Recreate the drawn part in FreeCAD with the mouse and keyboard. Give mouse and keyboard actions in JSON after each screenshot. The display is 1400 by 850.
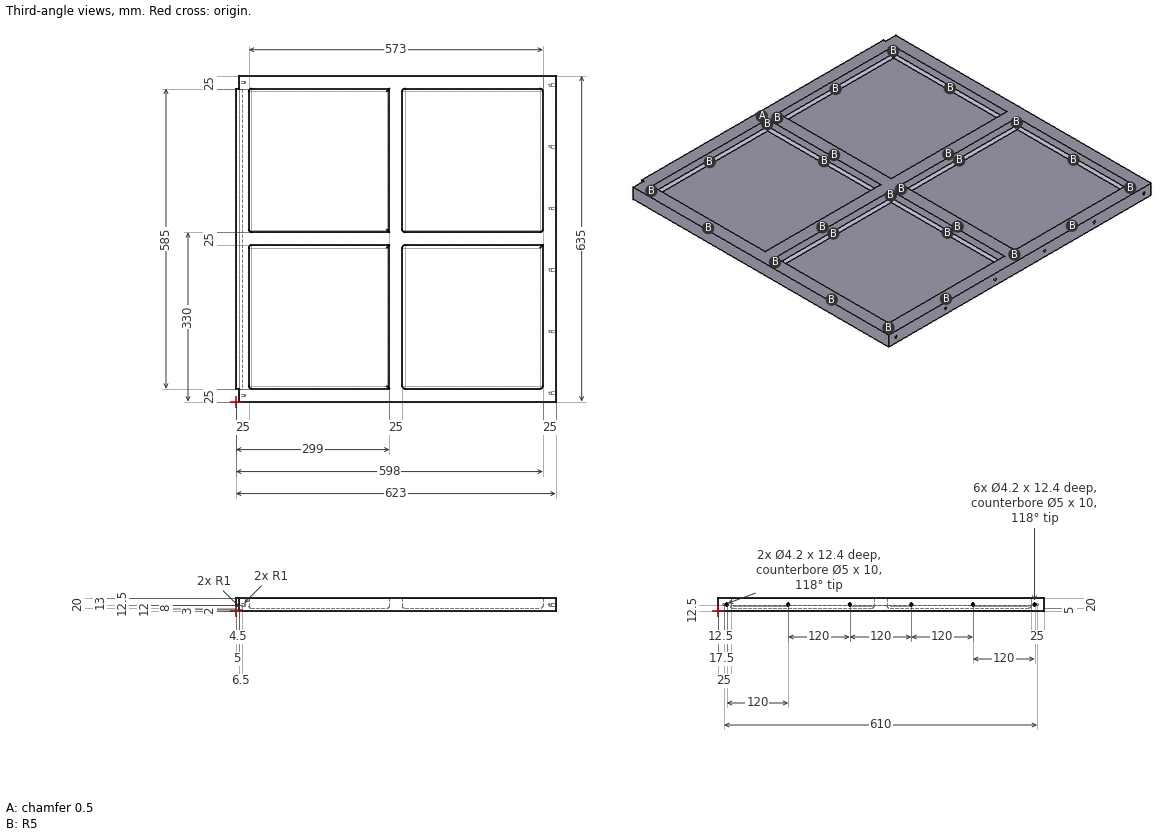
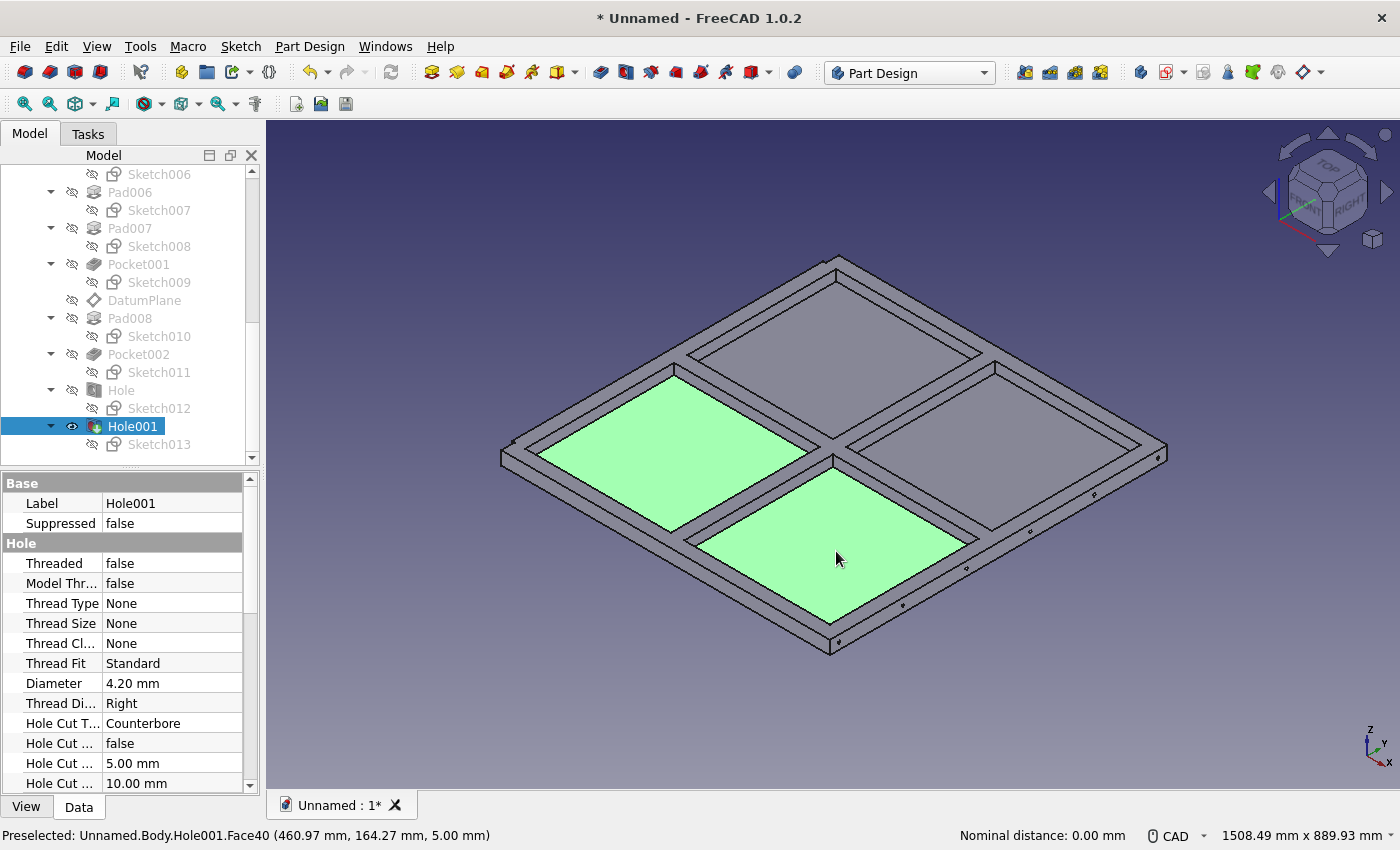
{"action": "left_click", "coordinate": [835, 365], "text": "ctrl"}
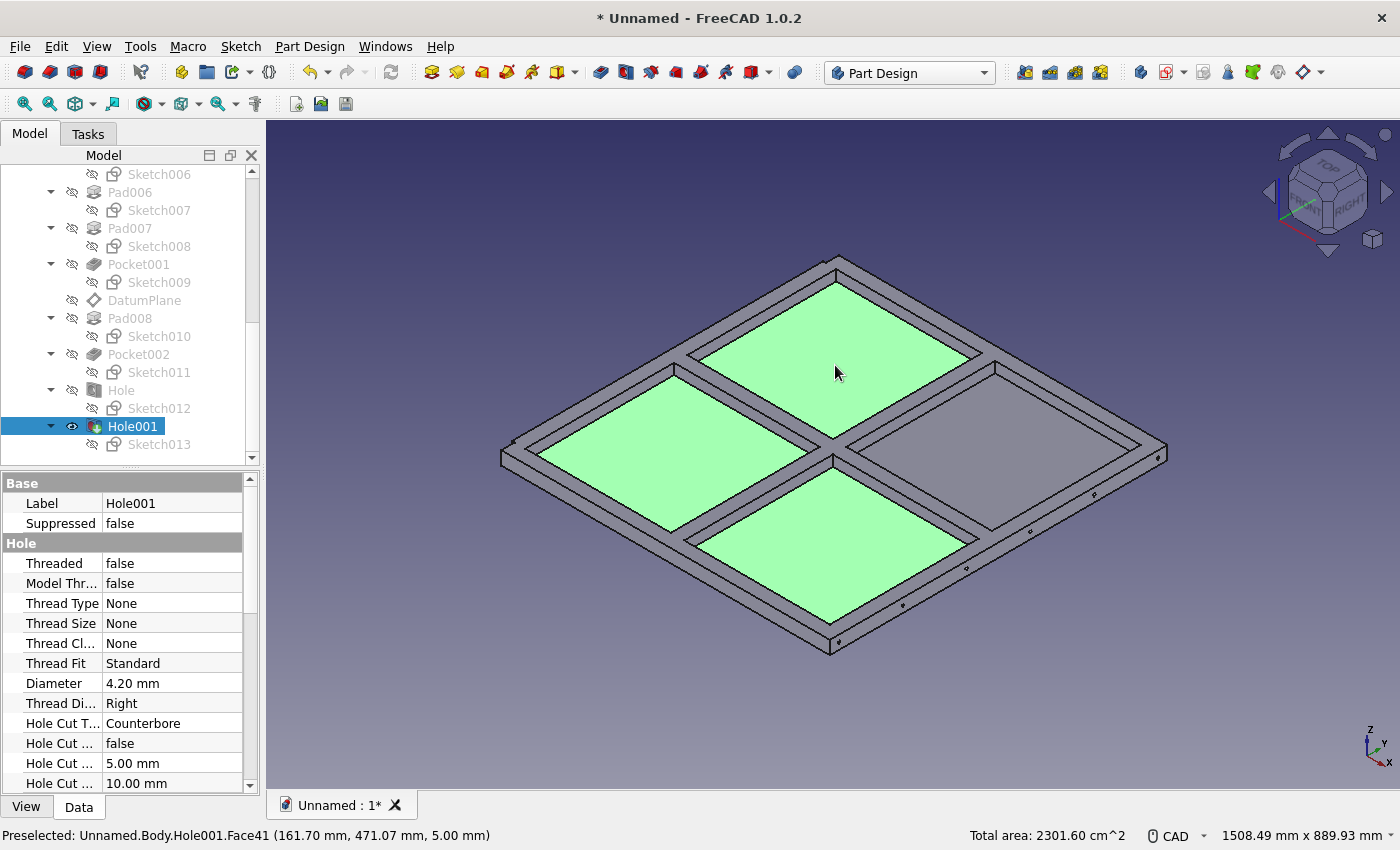
{"action": "left_click", "coordinate": [994, 457], "text": "ctrl"}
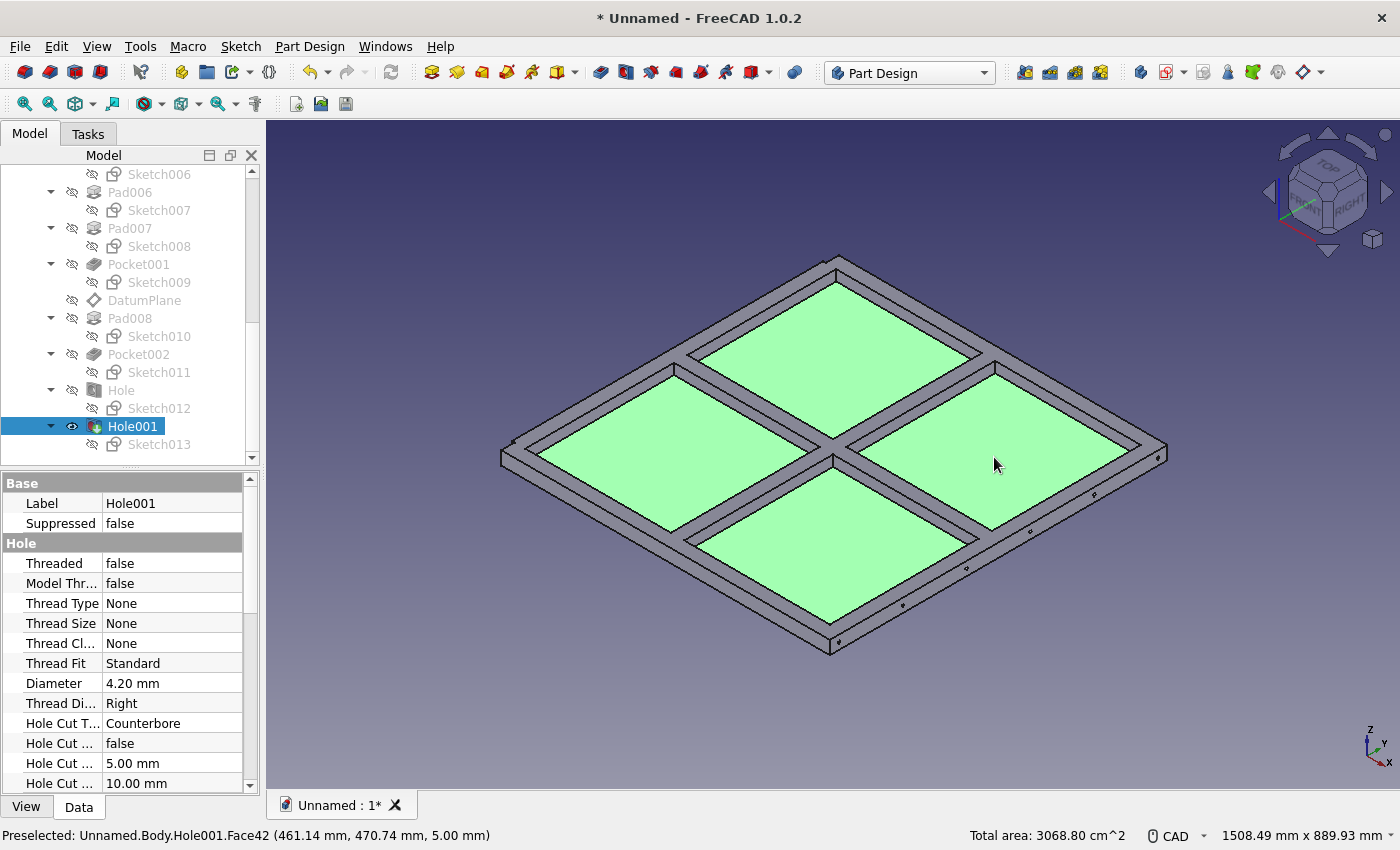
{"action": "scroll", "coordinate": [830, 630], "scroll_direction": "up", "scroll_amount": 5}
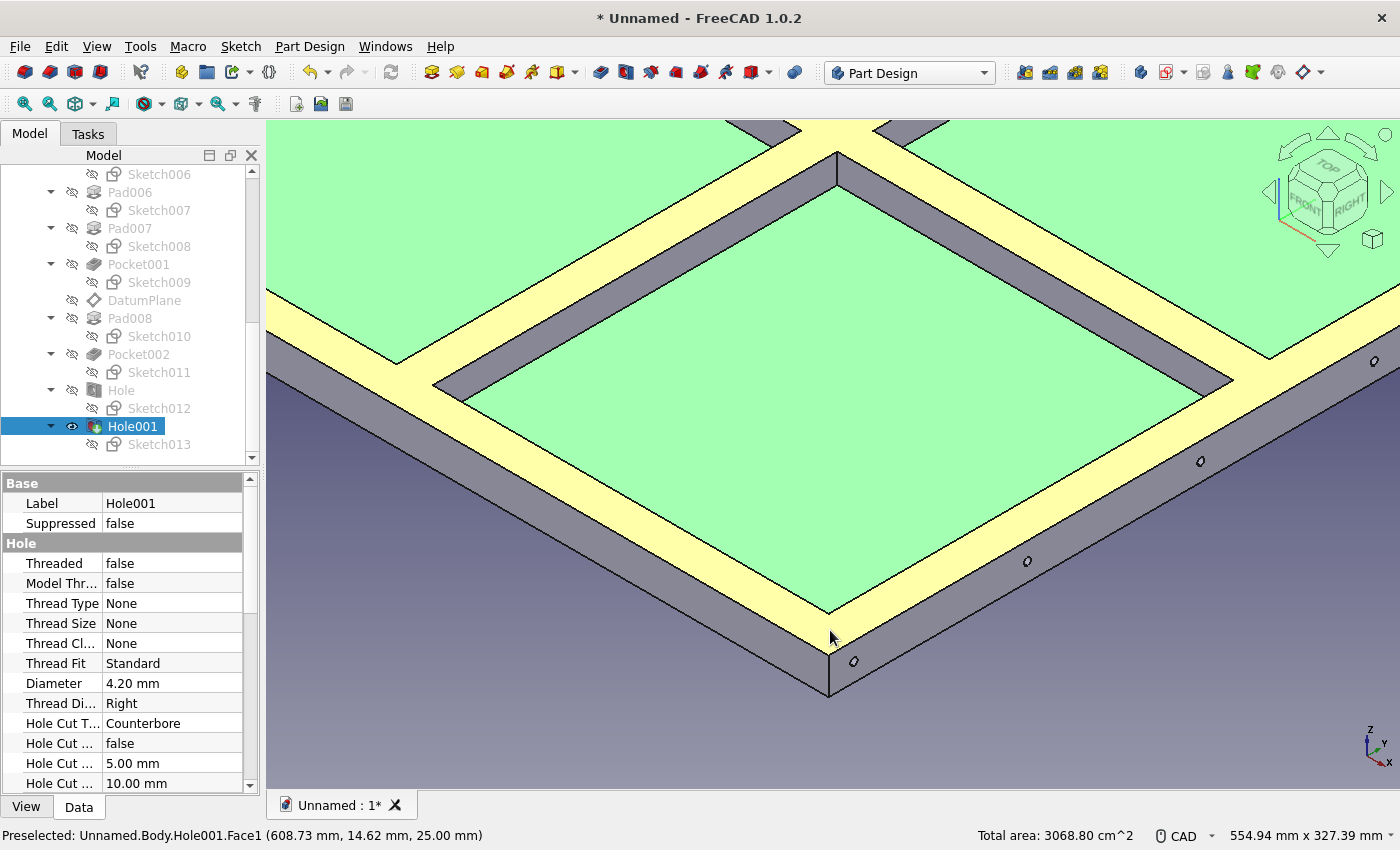
{"action": "left_click", "coordinate": [25, 104]}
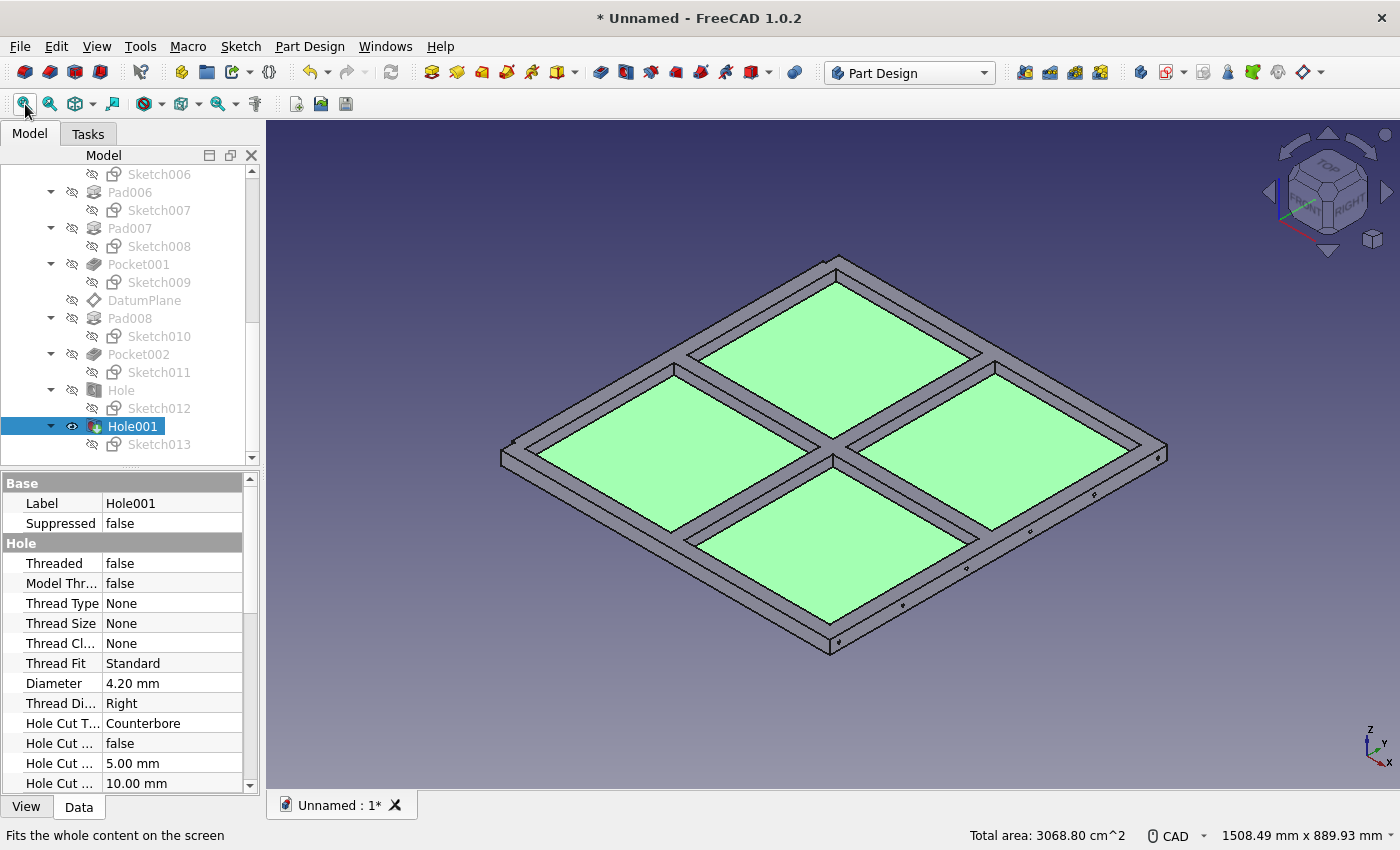
{"action": "key", "text": "2"}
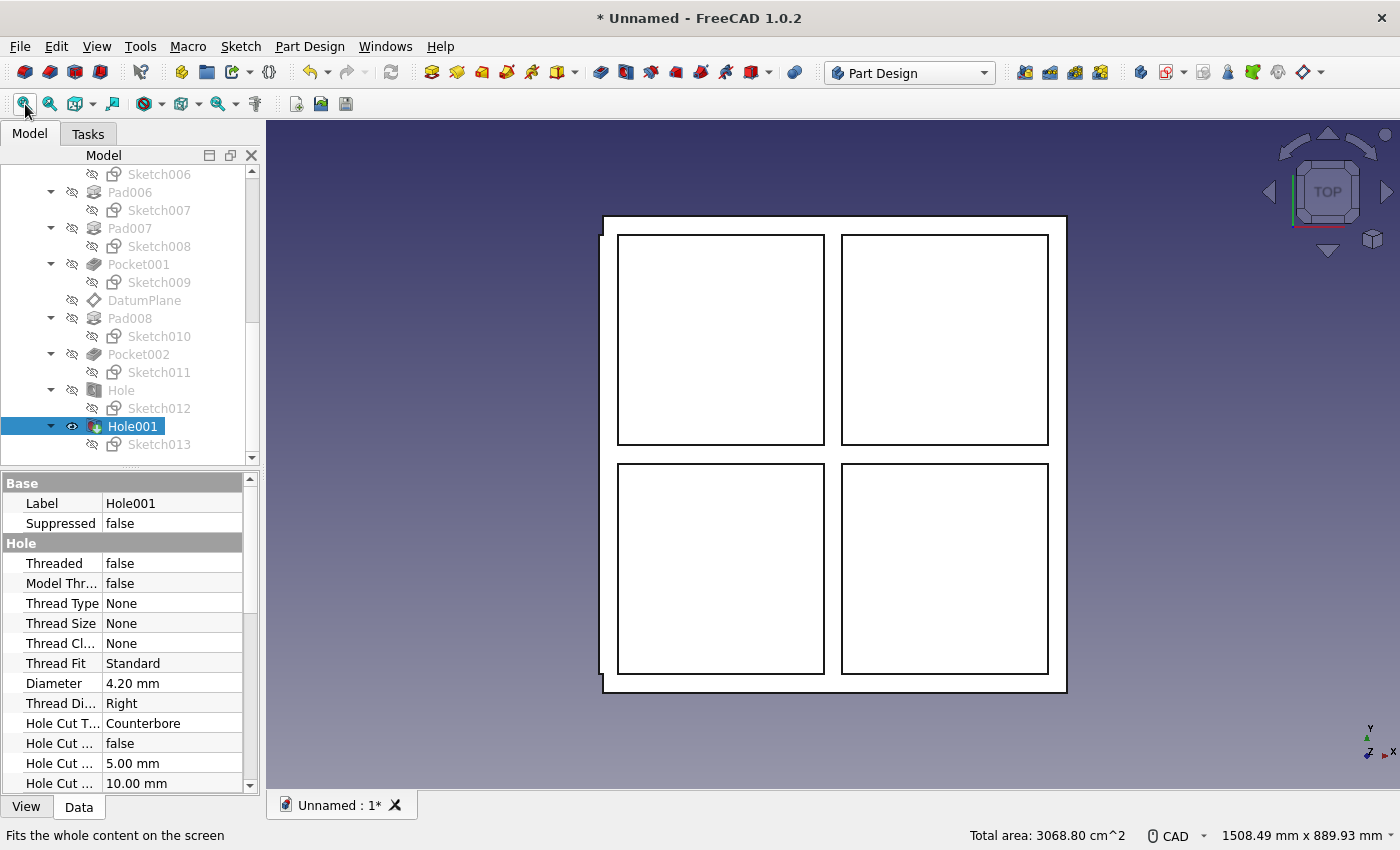
{"action": "scroll", "coordinate": [1048, 673], "scroll_direction": "up", "scroll_amount": 5}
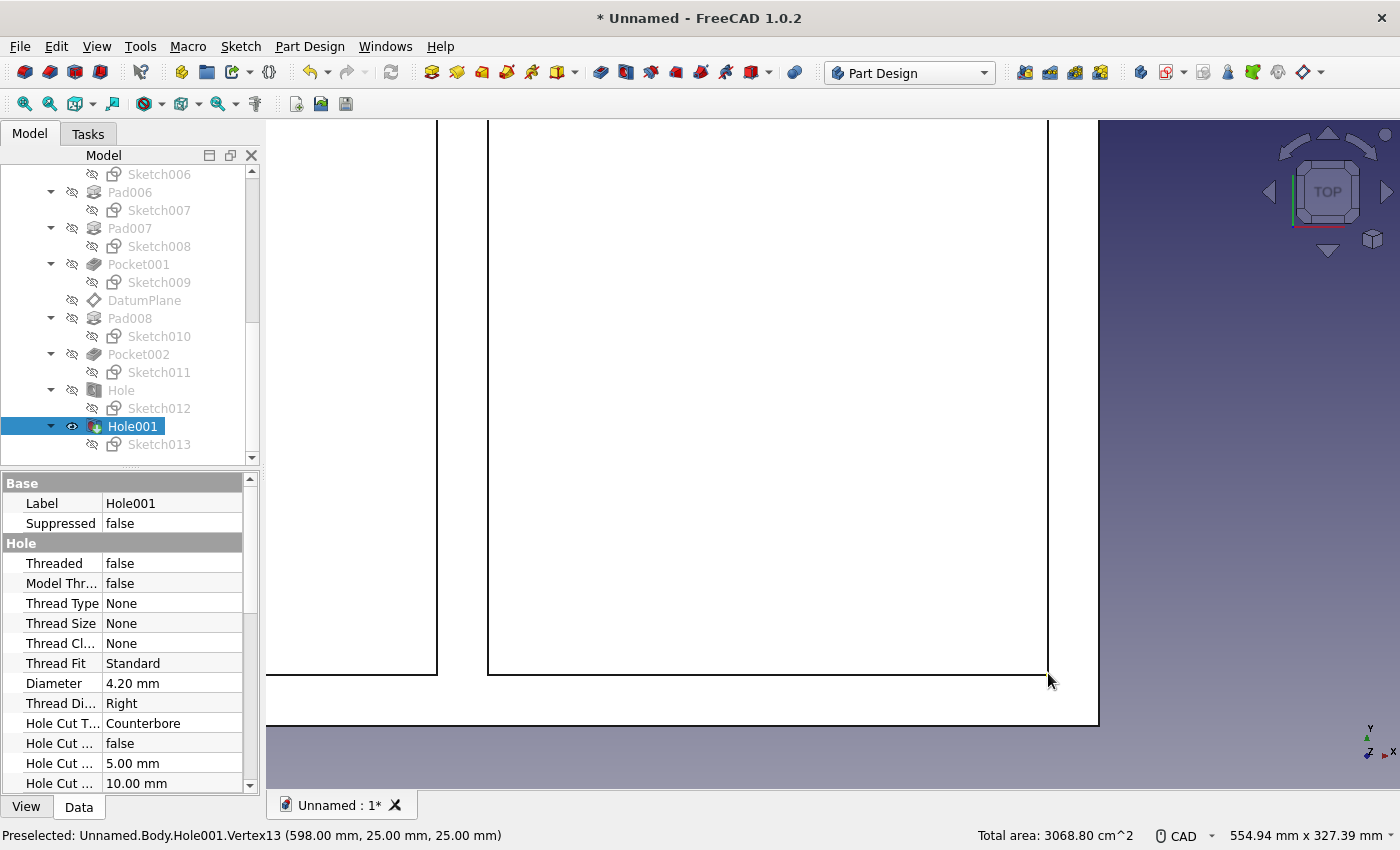
{"action": "left_click", "coordinate": [25, 104]}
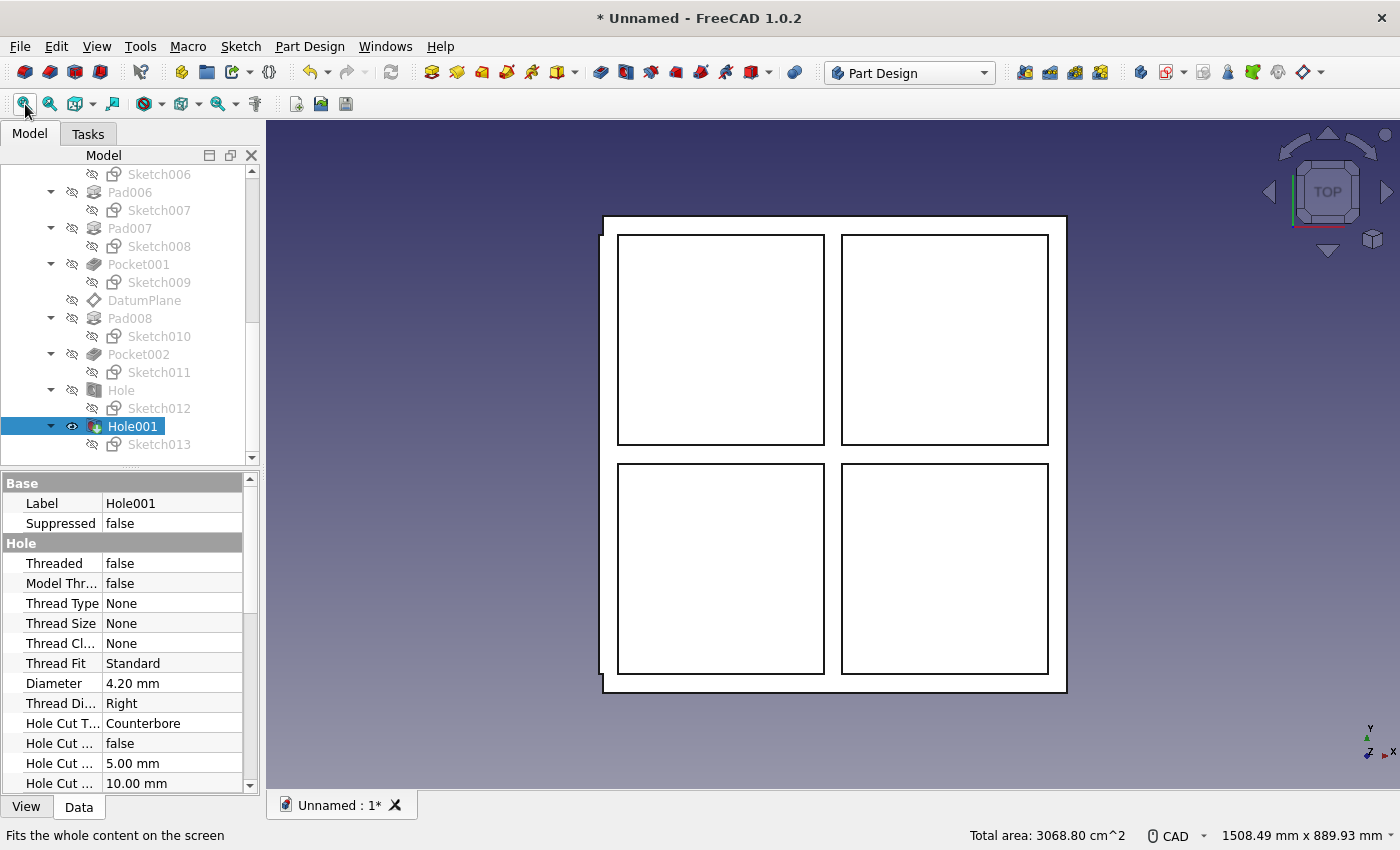
{"action": "key", "text": "1"}